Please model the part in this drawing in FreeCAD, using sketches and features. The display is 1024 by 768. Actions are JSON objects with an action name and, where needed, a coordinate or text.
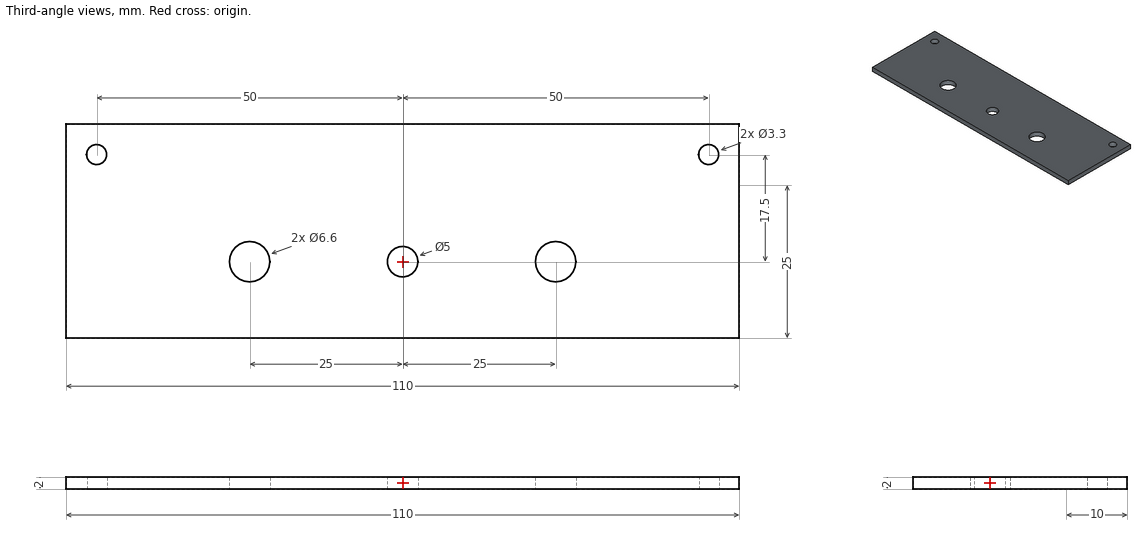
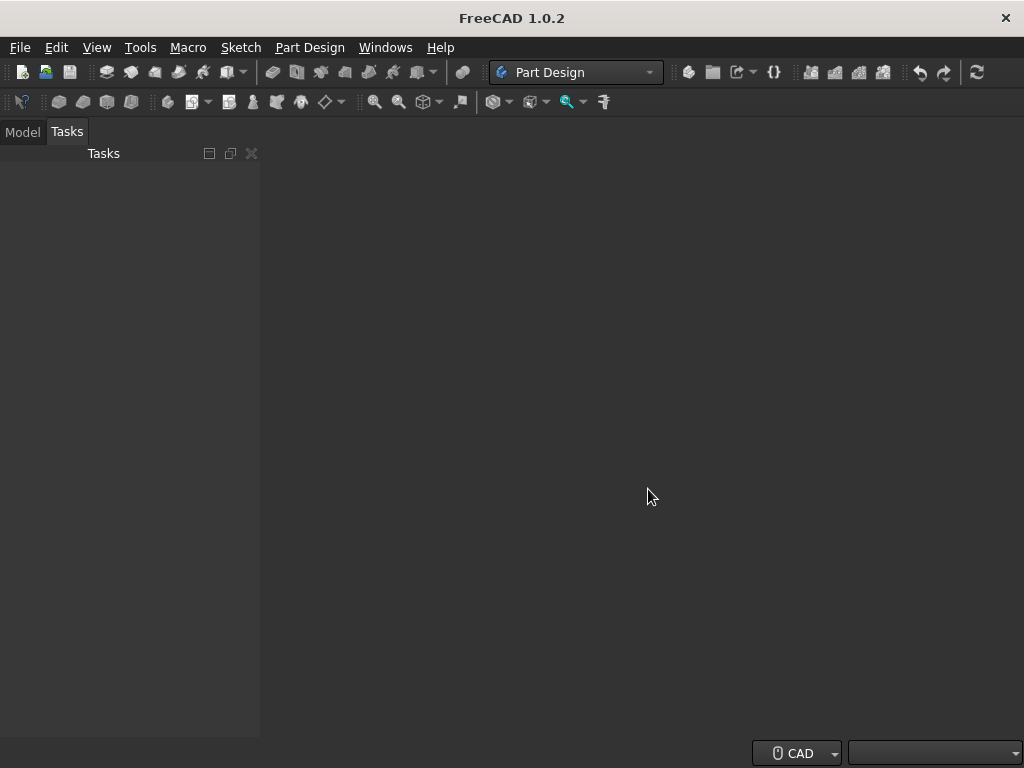
{"action": "left_click", "coordinate": [22, 72]}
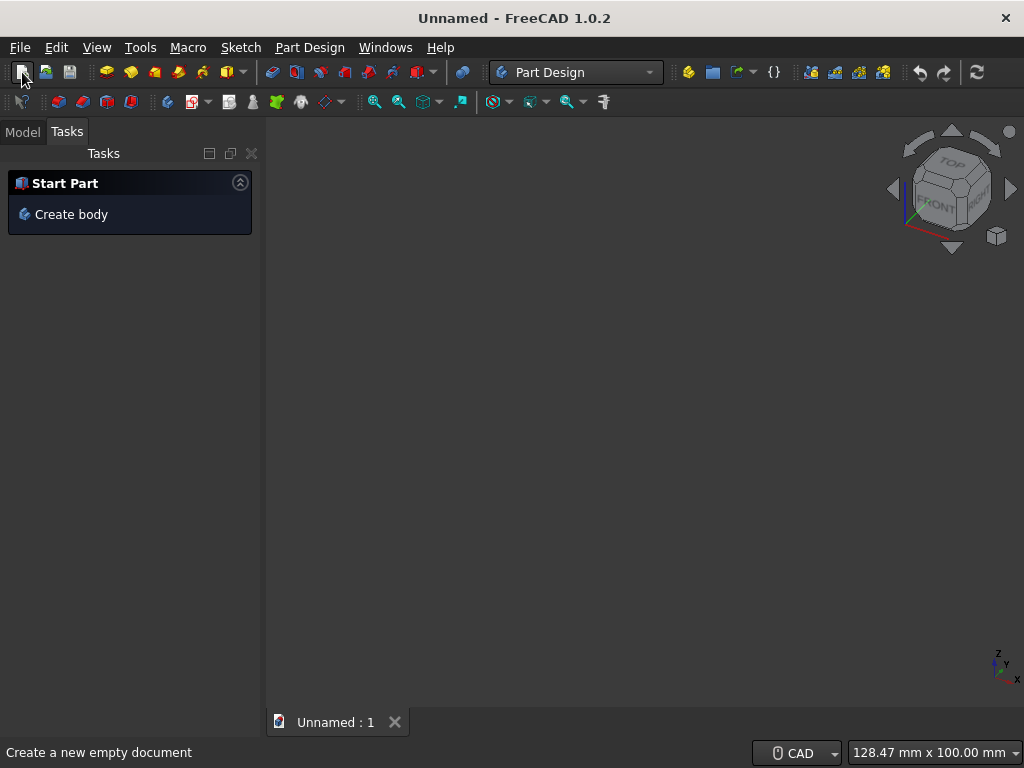
{"action": "left_click", "coordinate": [192, 102]}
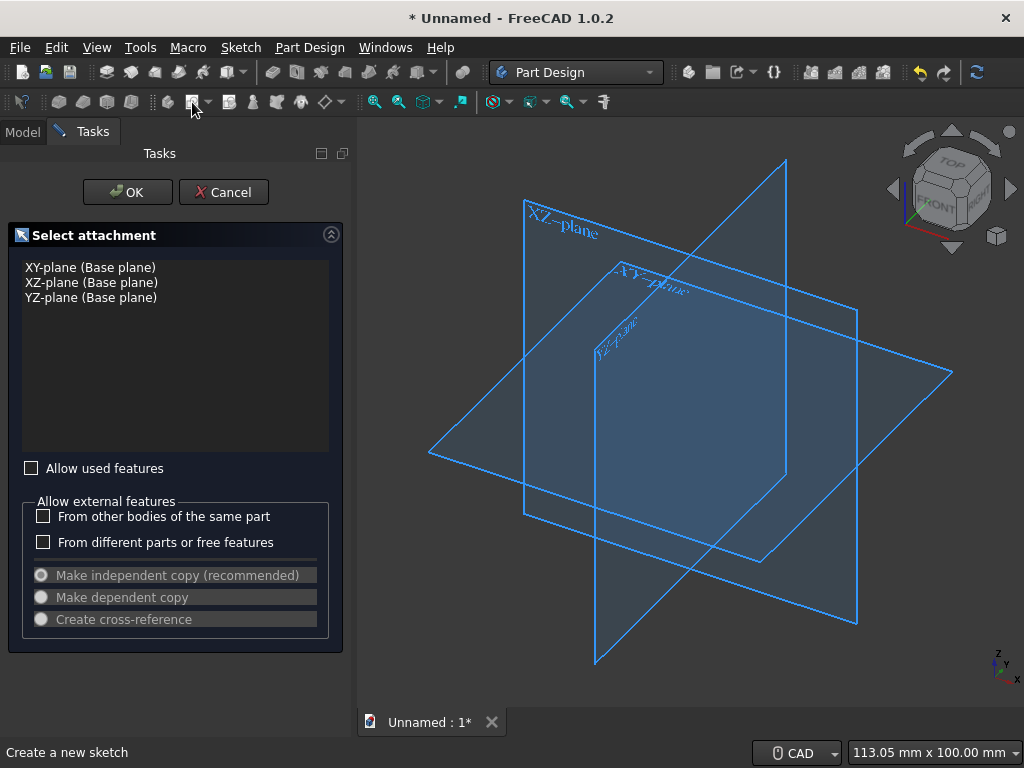
{"action": "left_click", "coordinate": [82, 268]}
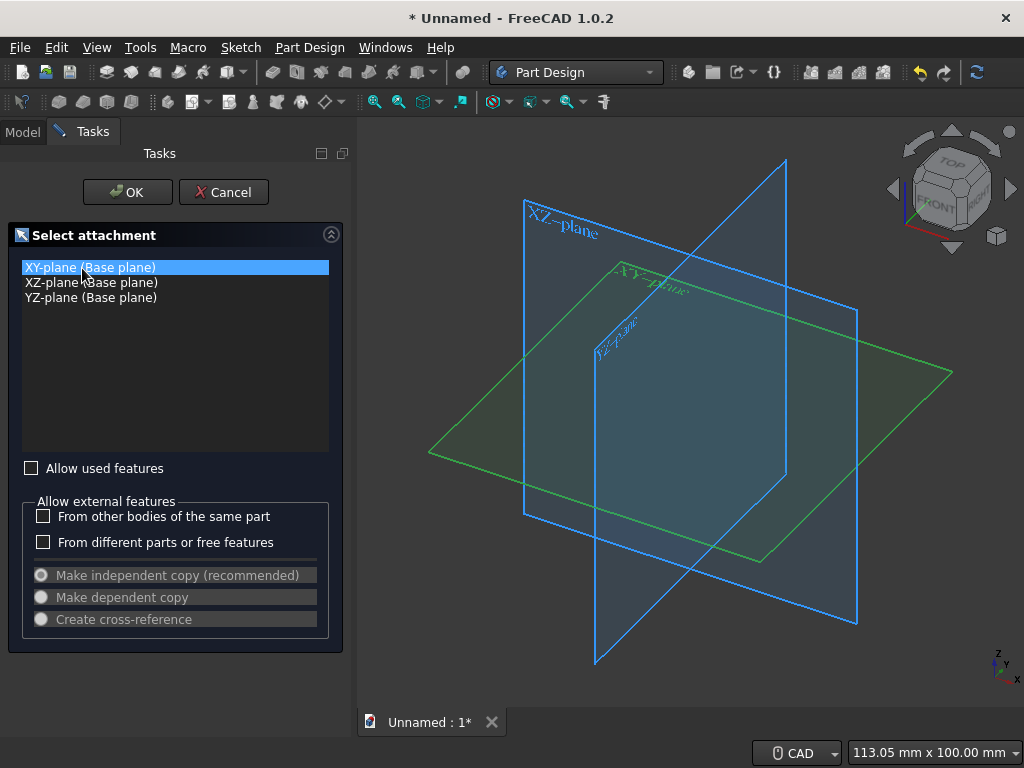
{"action": "left_click", "coordinate": [128, 192]}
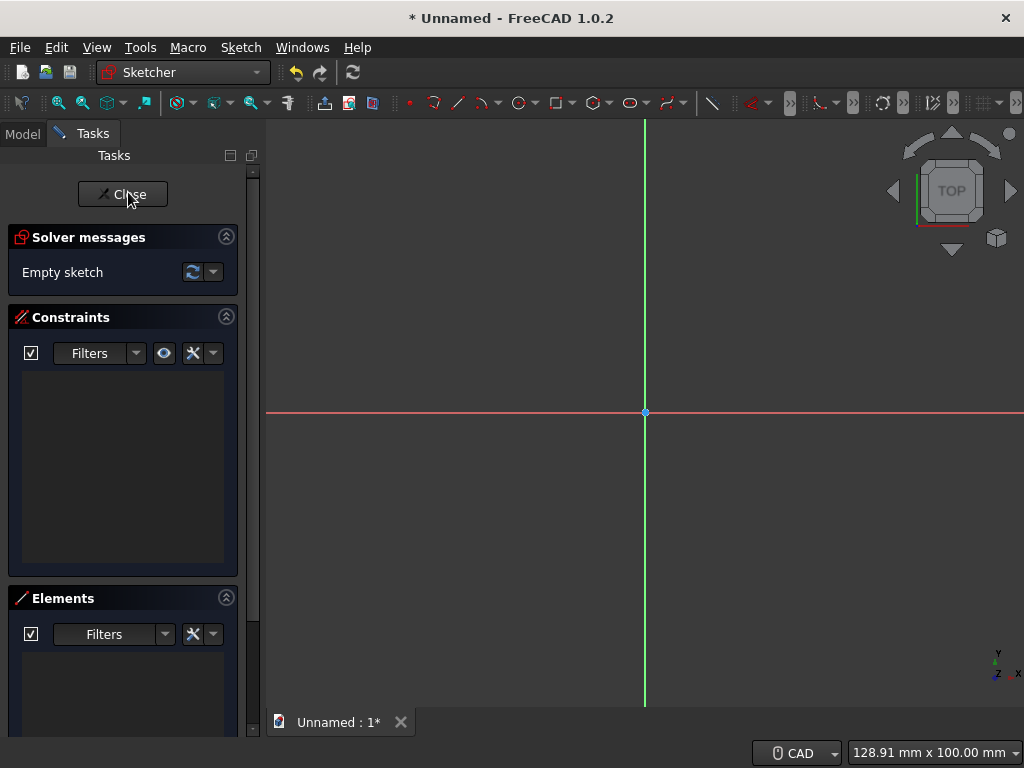
{"action": "scroll", "coordinate": [437, 413], "scroll_direction": "down", "scroll_amount": 2}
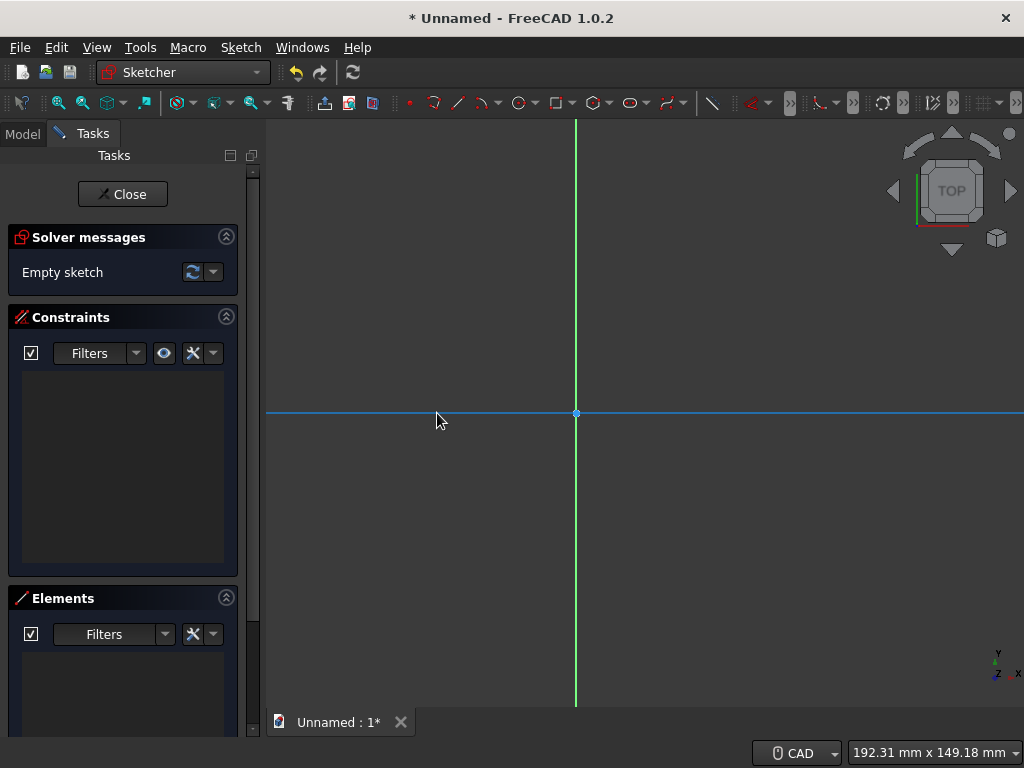
{"action": "left_click", "coordinate": [574, 104]}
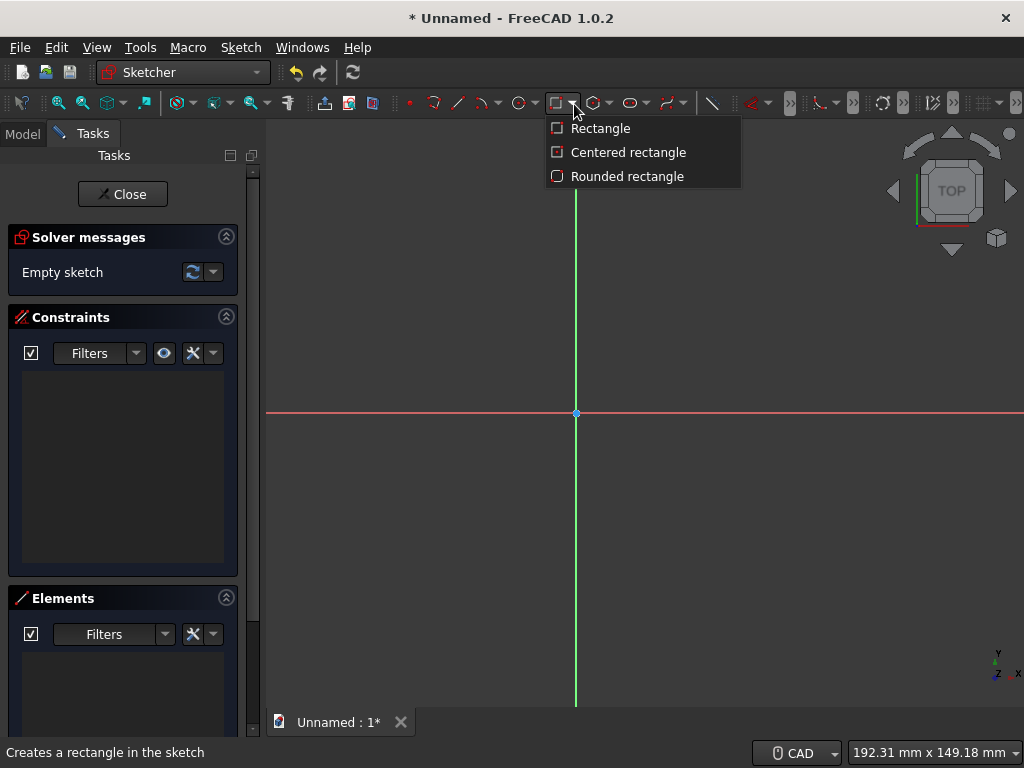
{"action": "left_click", "coordinate": [644, 152]}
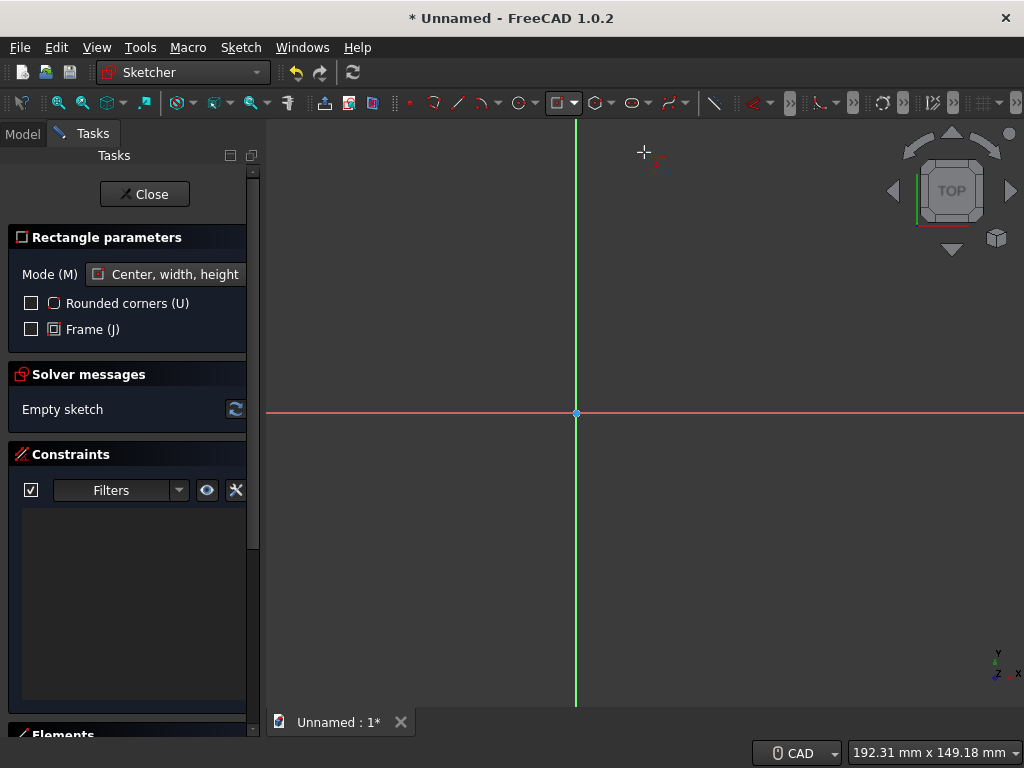
{"action": "left_click", "coordinate": [577, 413]}
{"action": "mouse_move", "coordinate": [793, 364]}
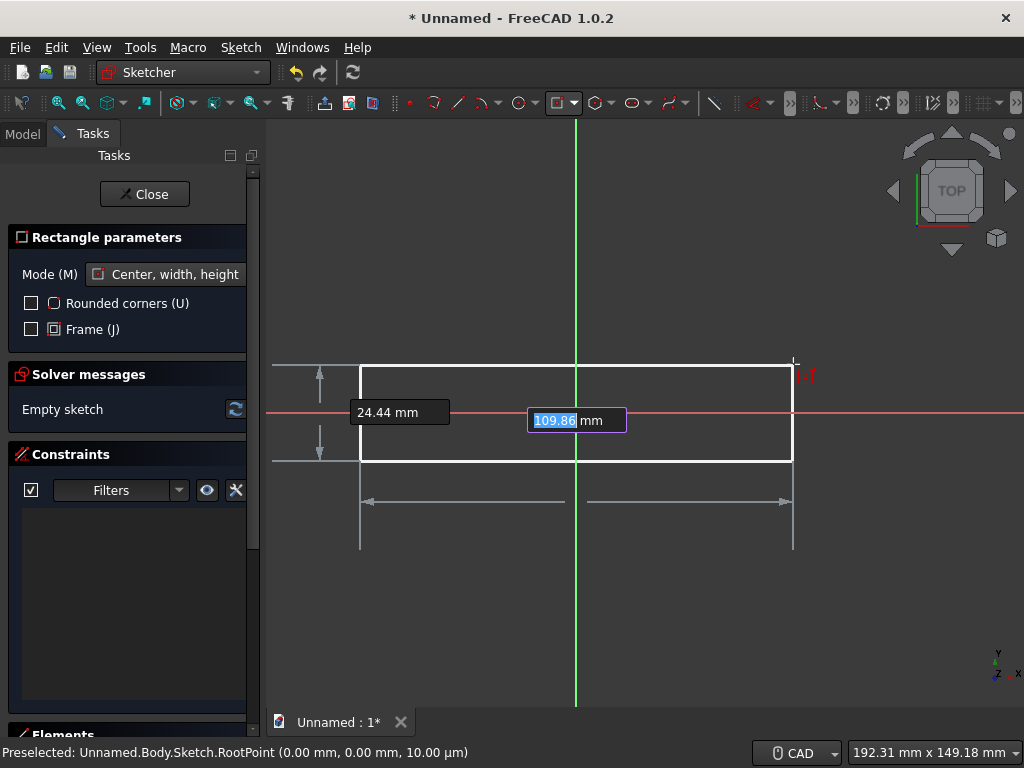
{"action": "type", "text": "110"}
{"action": "key", "text": "Tab"}
{"action": "type", "text": "25"}
{"action": "key", "text": "Return"}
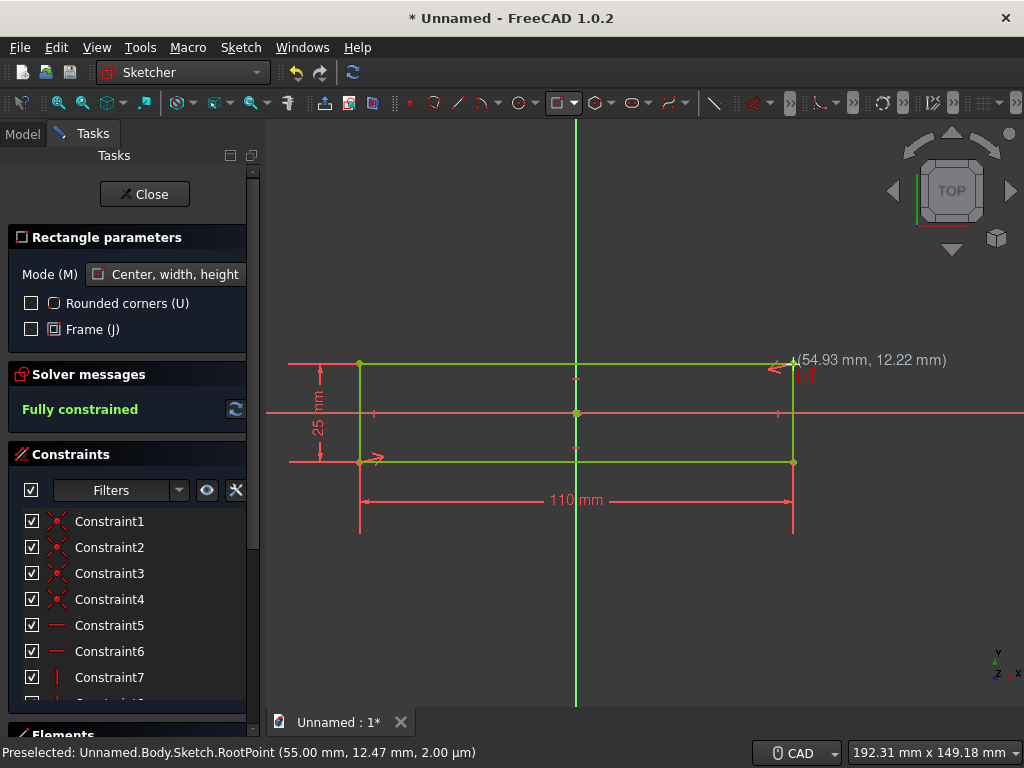
{"action": "left_click", "coordinate": [520, 104]}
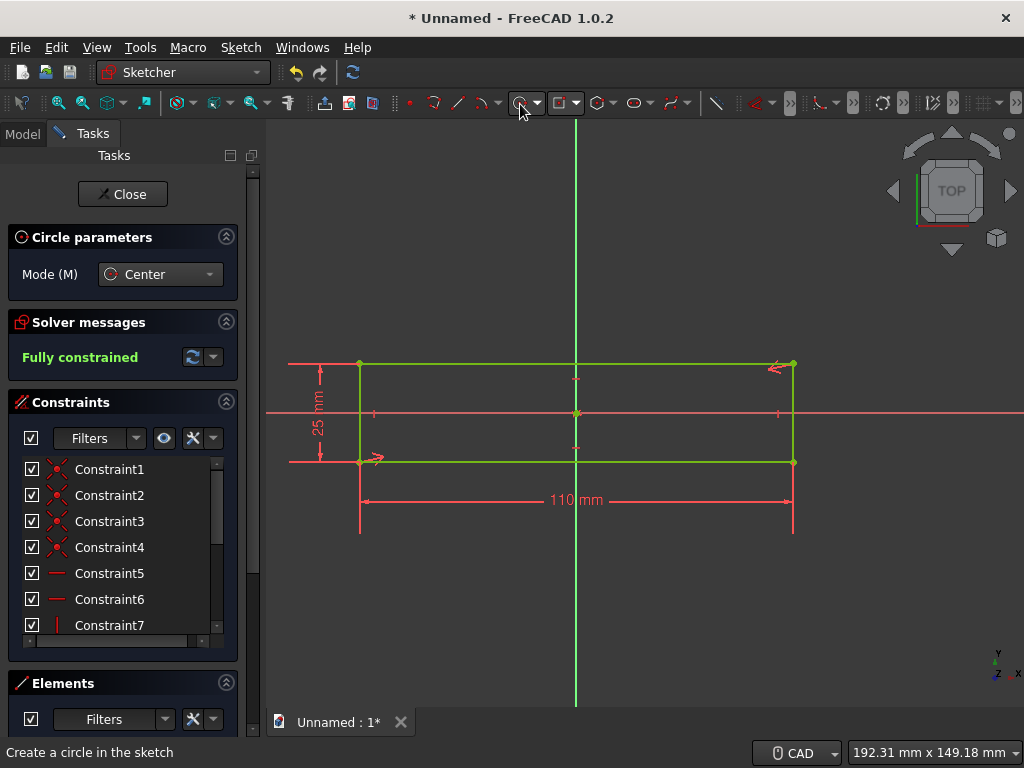
{"action": "scroll", "coordinate": [478, 413], "scroll_direction": "up", "scroll_amount": 3}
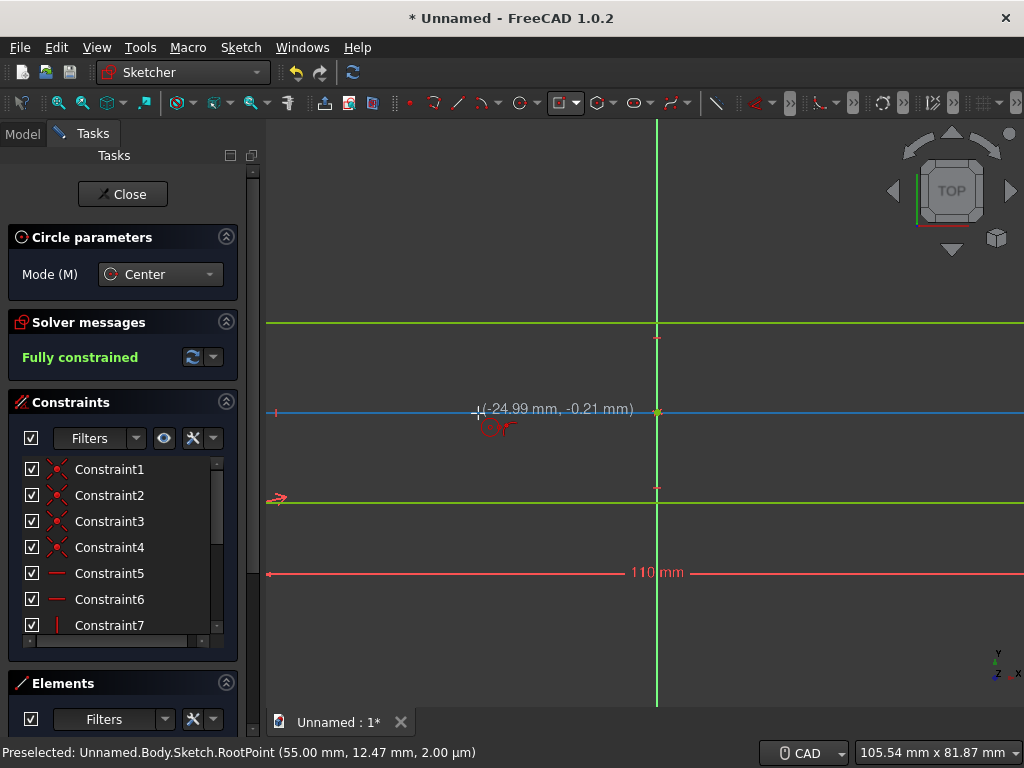
{"action": "left_click", "coordinate": [478, 413]}
{"action": "mouse_move", "coordinate": [494, 396]}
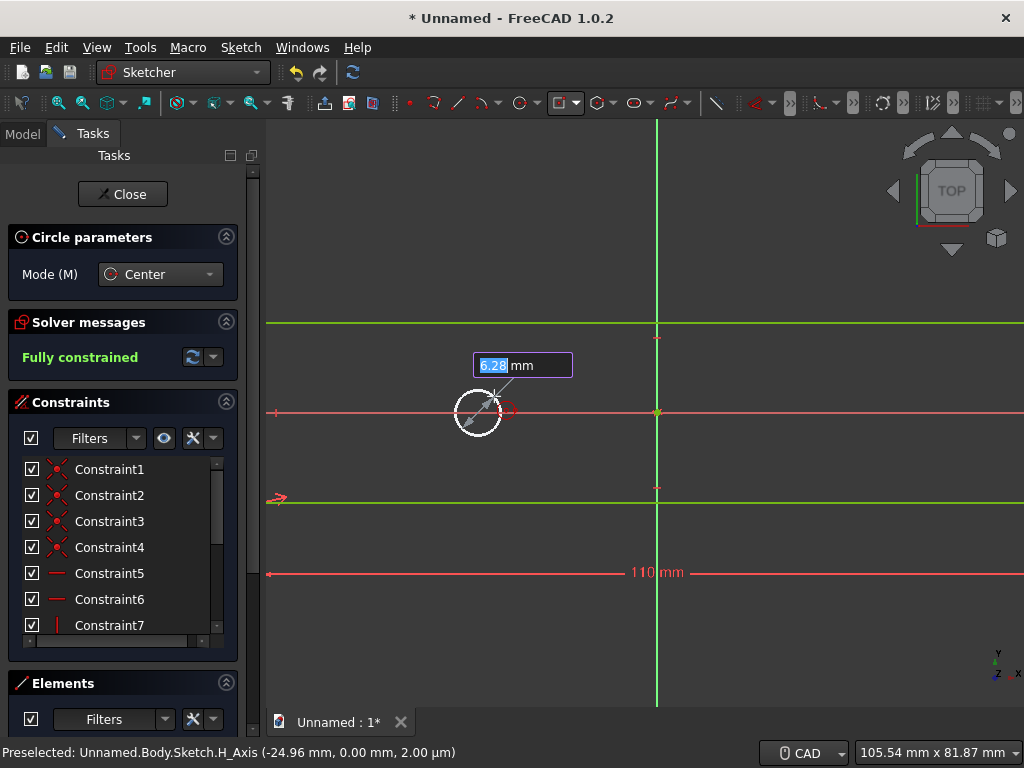
{"action": "type", "text": "6.6"}
{"action": "key", "text": "Return"}